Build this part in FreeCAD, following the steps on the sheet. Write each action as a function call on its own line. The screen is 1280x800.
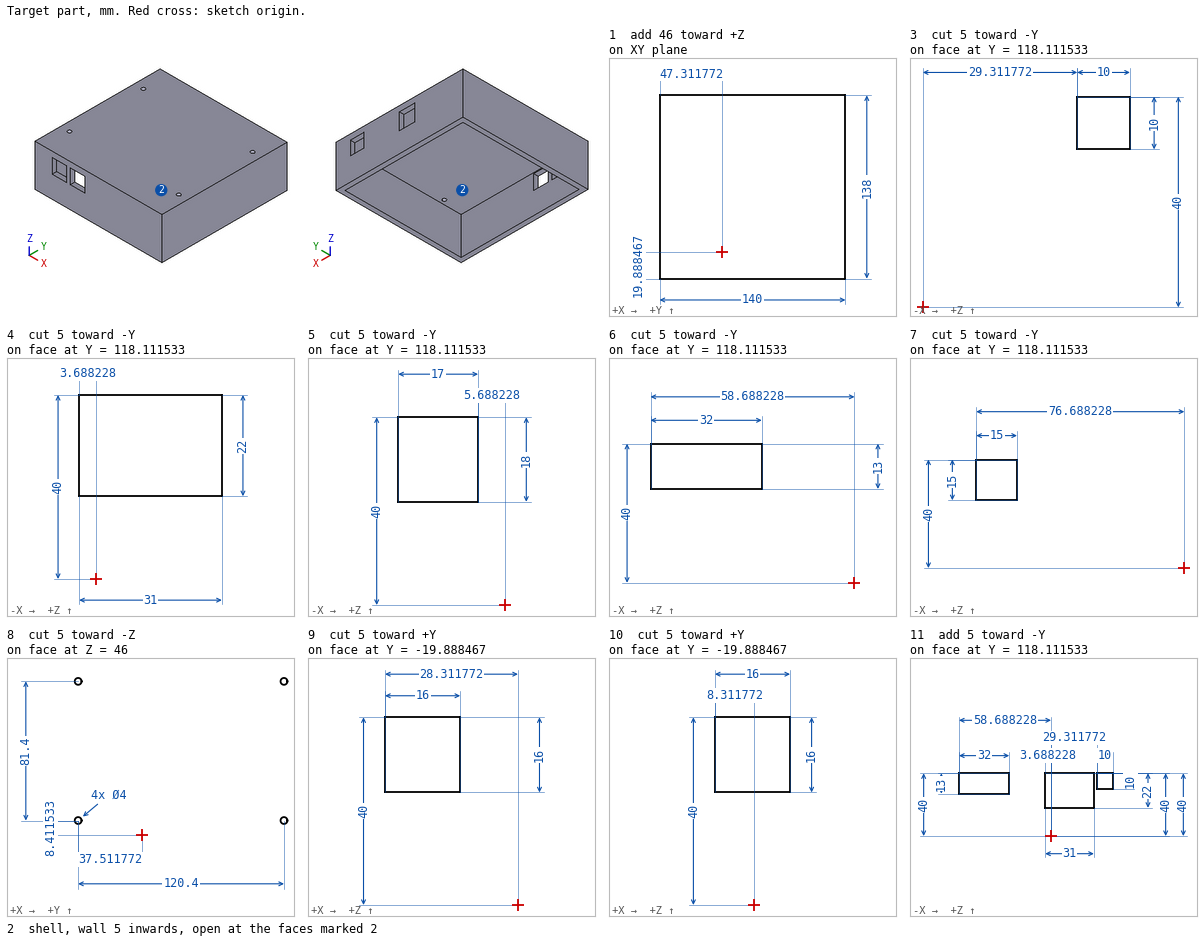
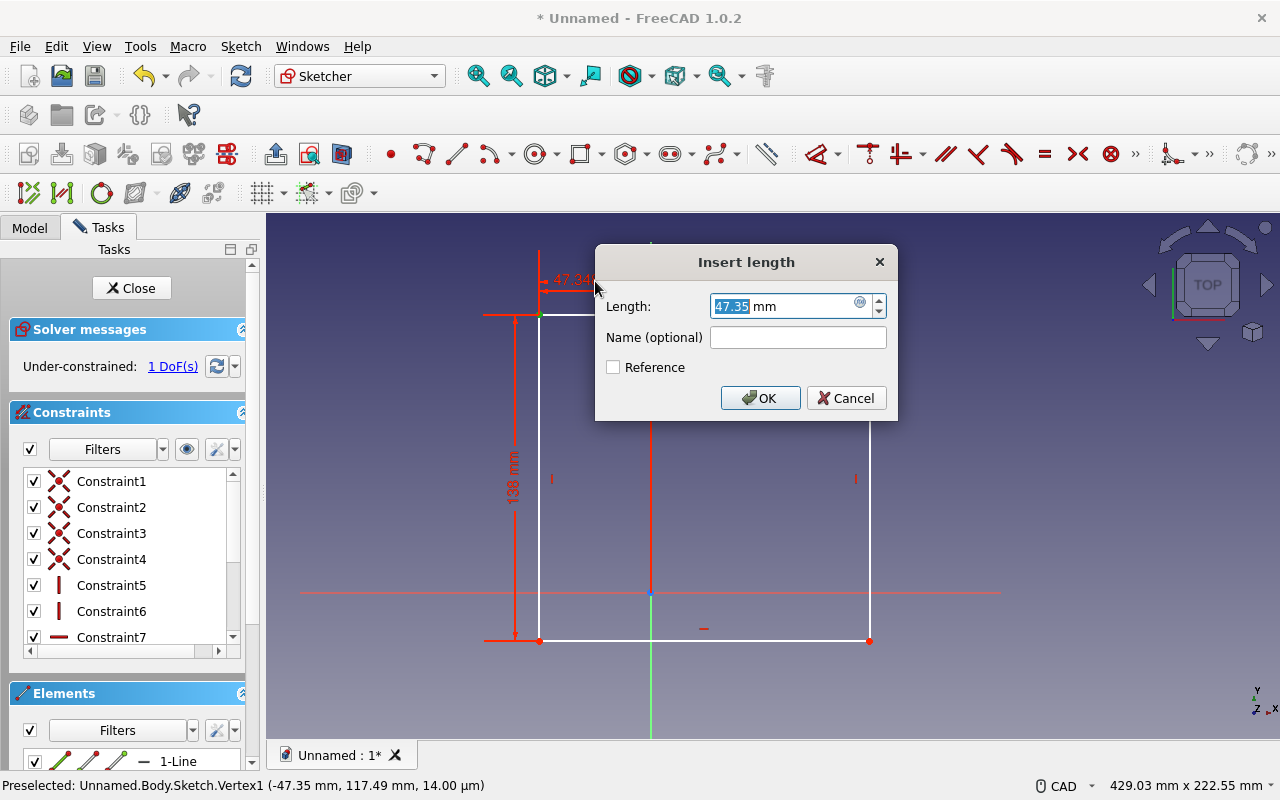
text(47.311772)
key(Return)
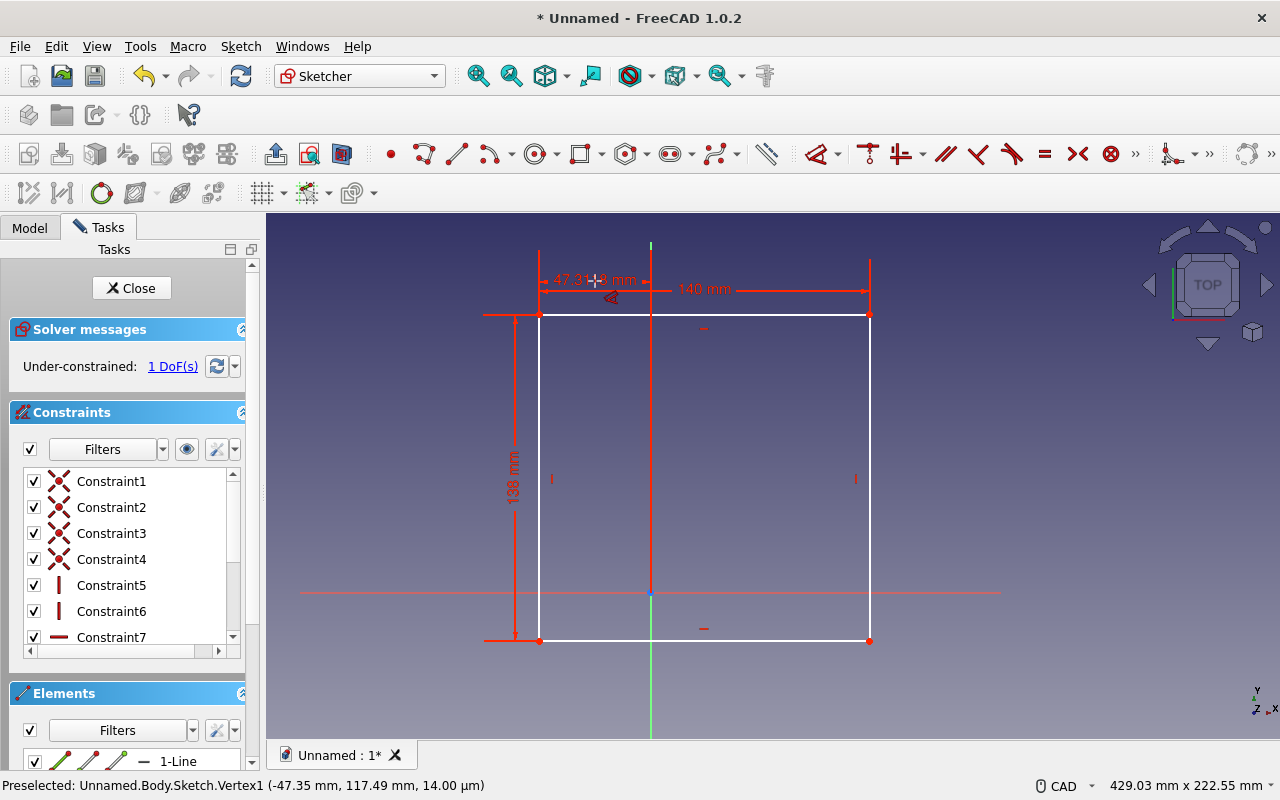
click(539, 641)
click(505, 617)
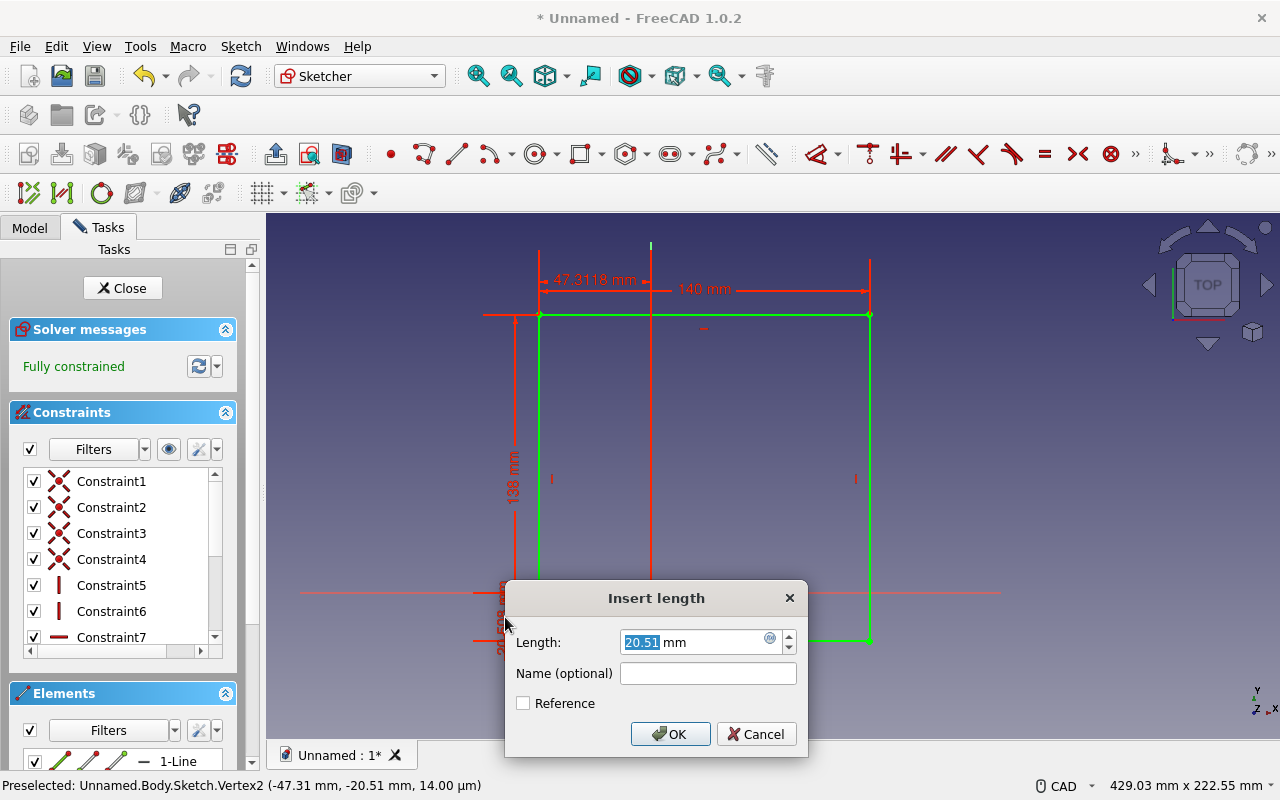
text(19.888467)
key(Return)
key(Escape)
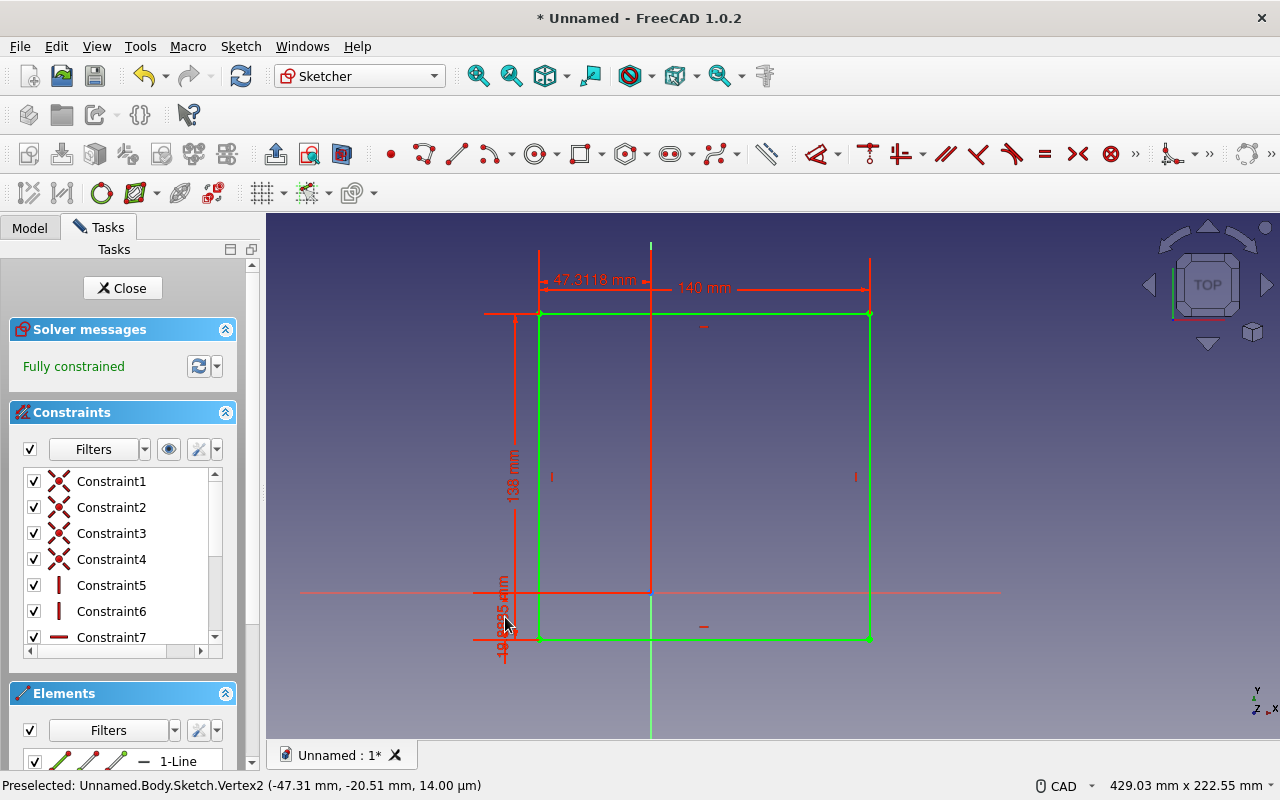
click(123, 288)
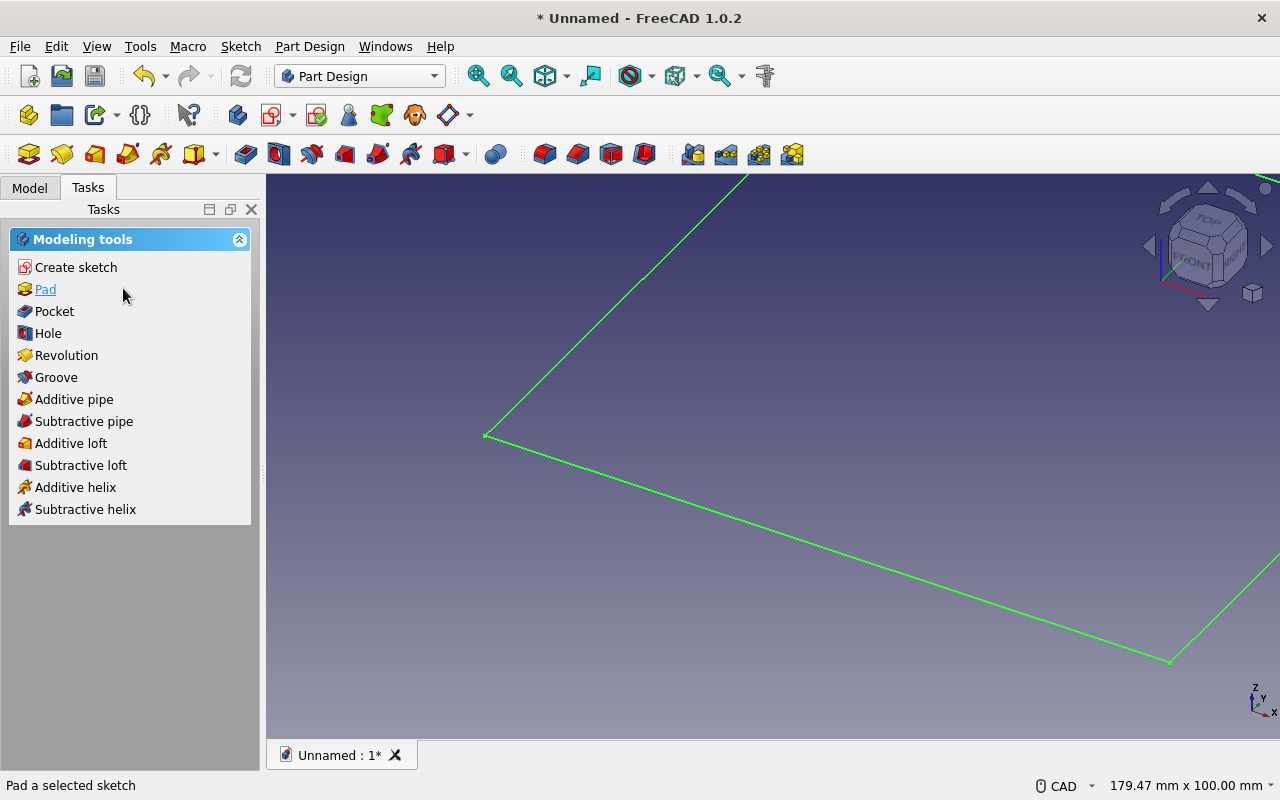
click(29, 154)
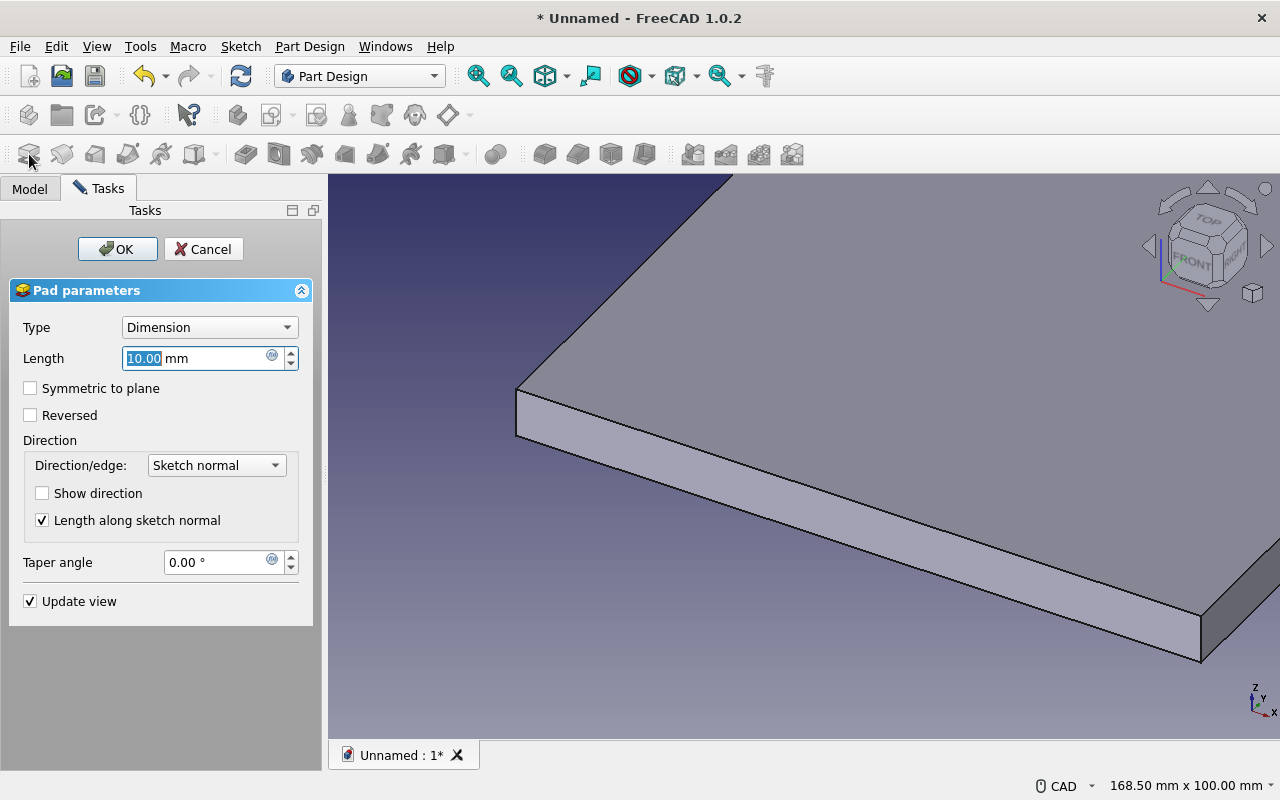
text(46)
key(Tab)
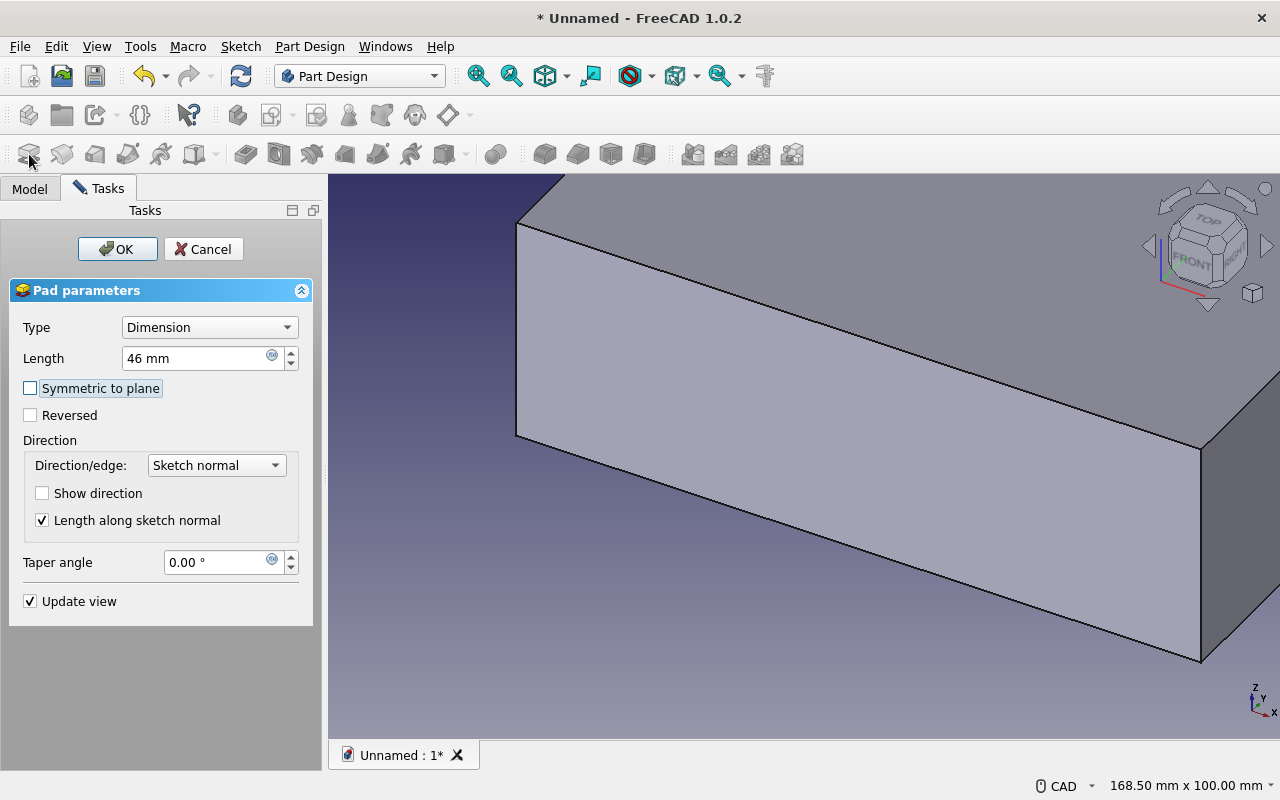
click(118, 249)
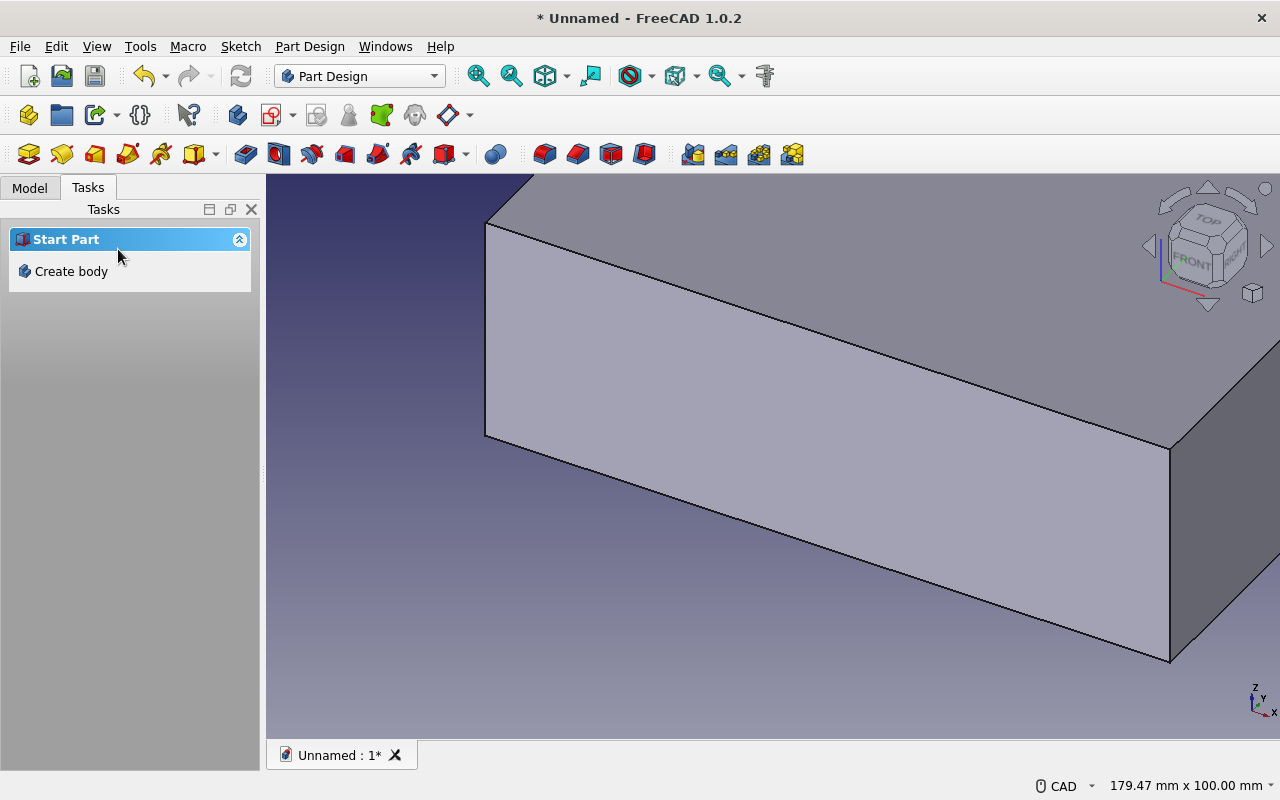
click(479, 76)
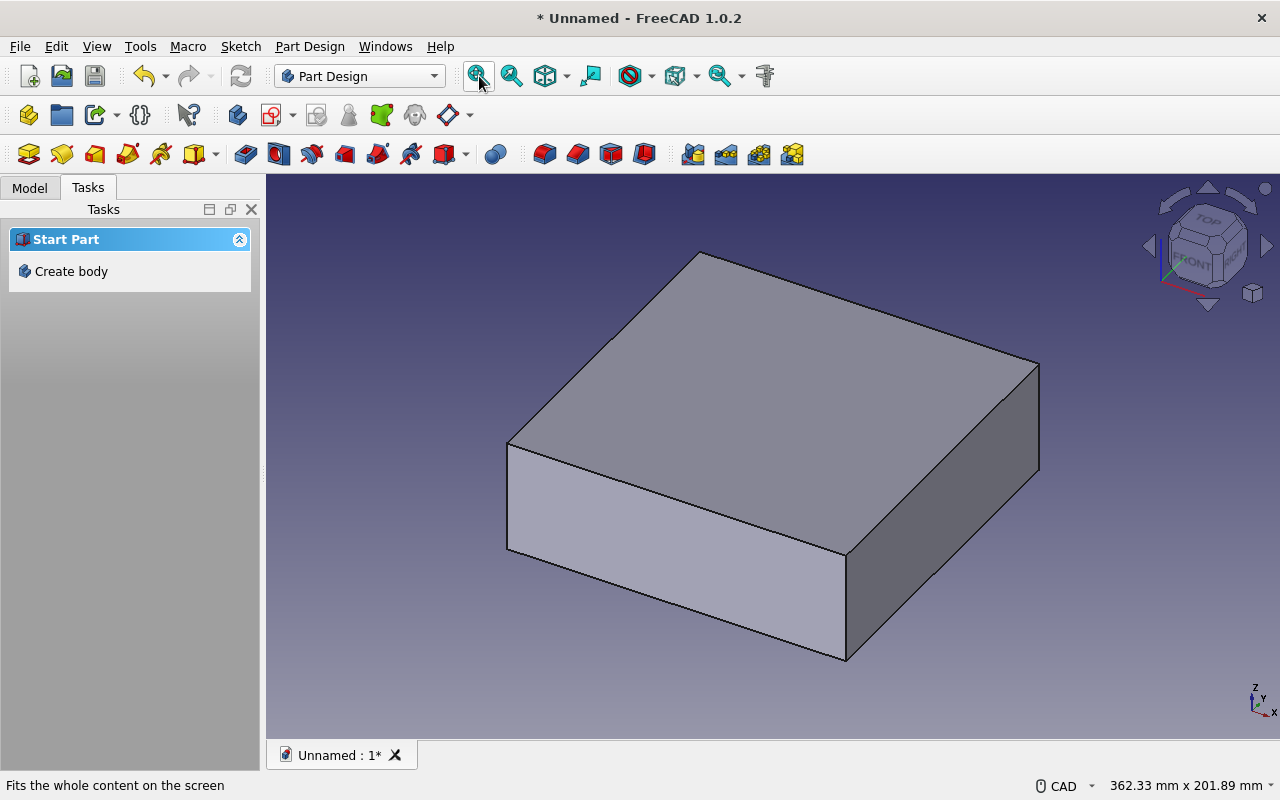
key(0)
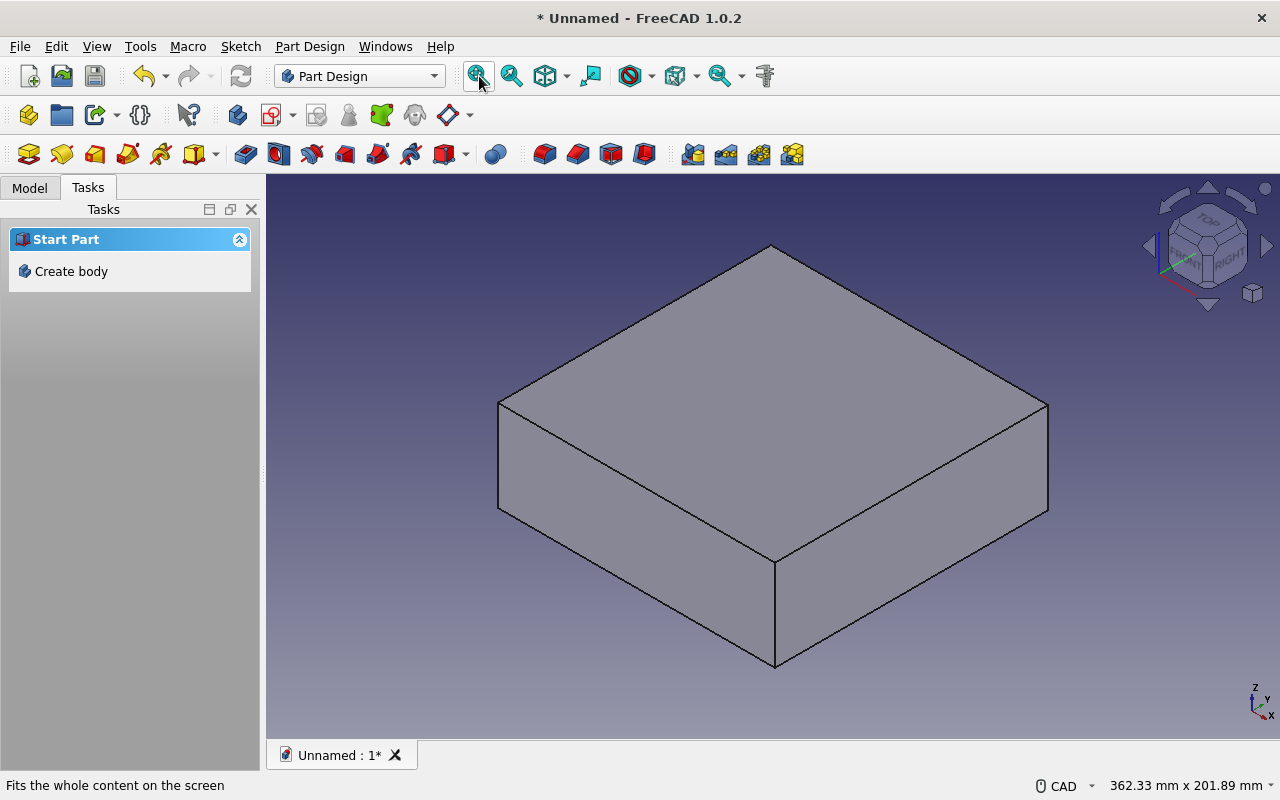
key(2)